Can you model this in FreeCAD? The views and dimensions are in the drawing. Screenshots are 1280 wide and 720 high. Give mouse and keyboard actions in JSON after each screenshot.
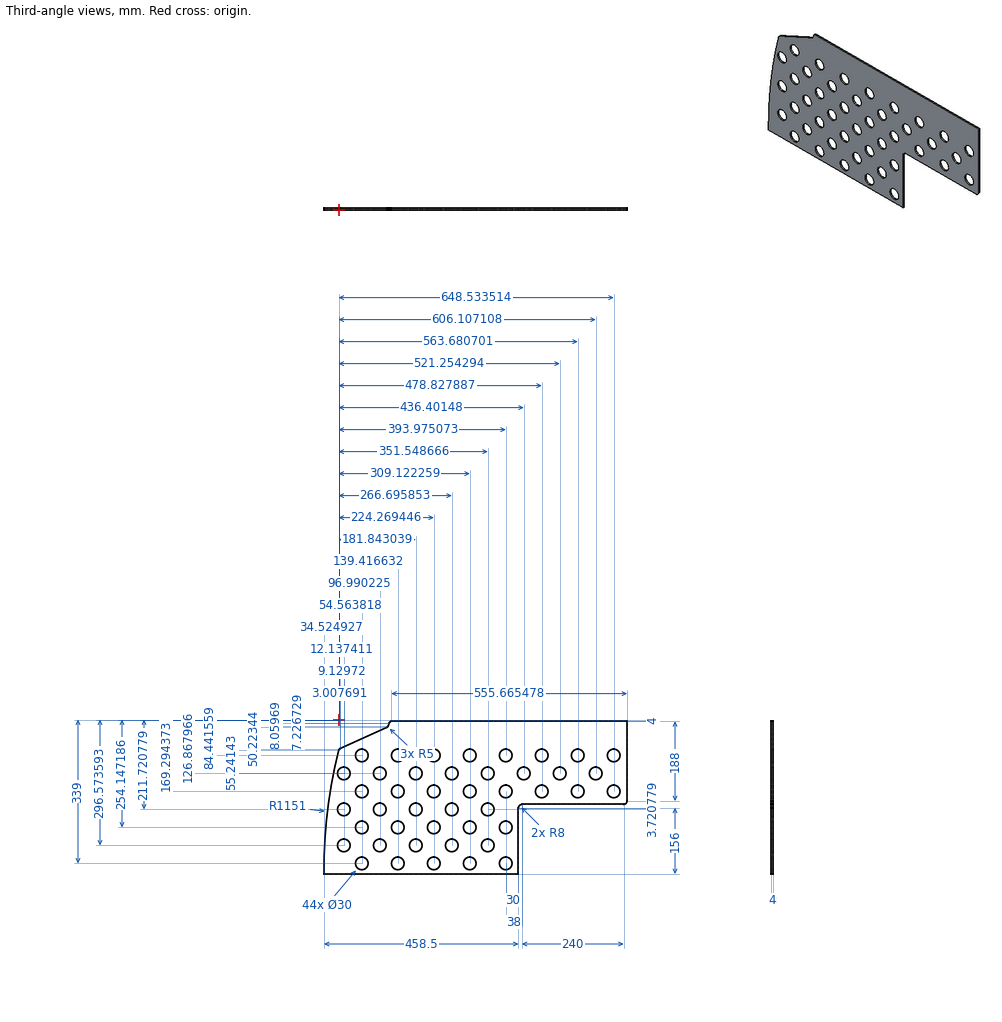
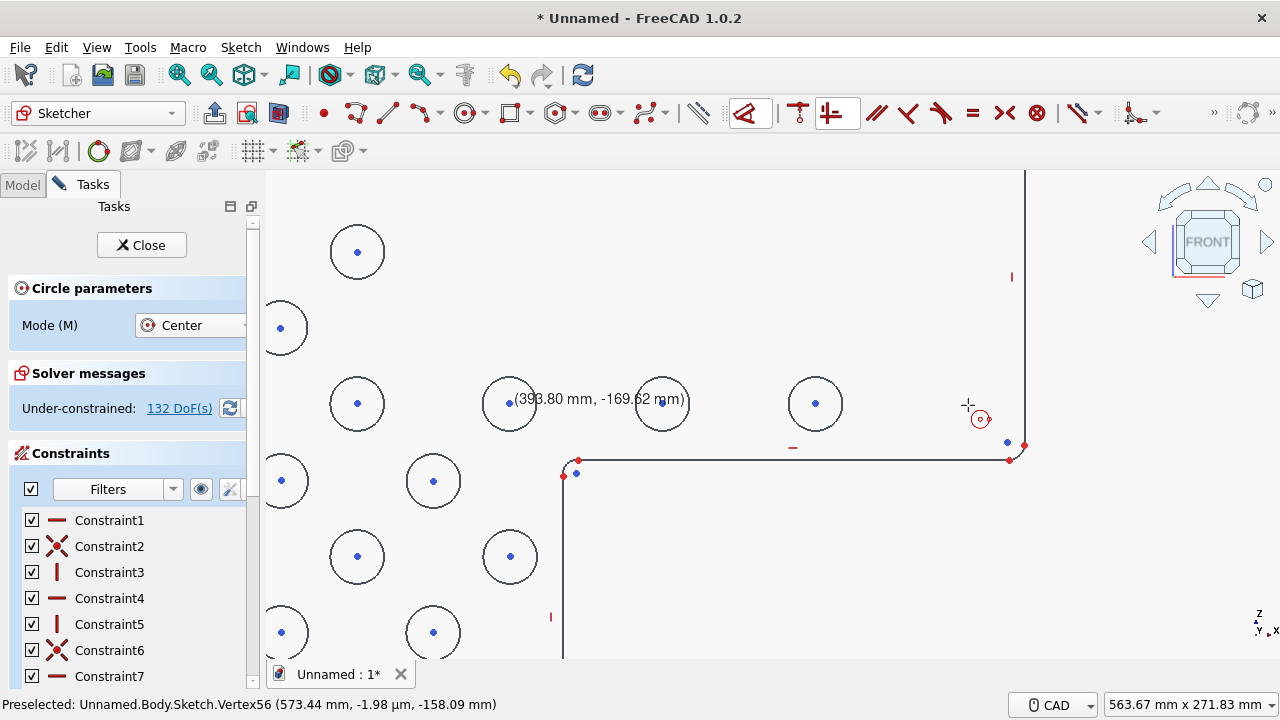
{"action": "left_click", "coordinate": [968, 403]}
{"action": "left_click", "coordinate": [987, 384]}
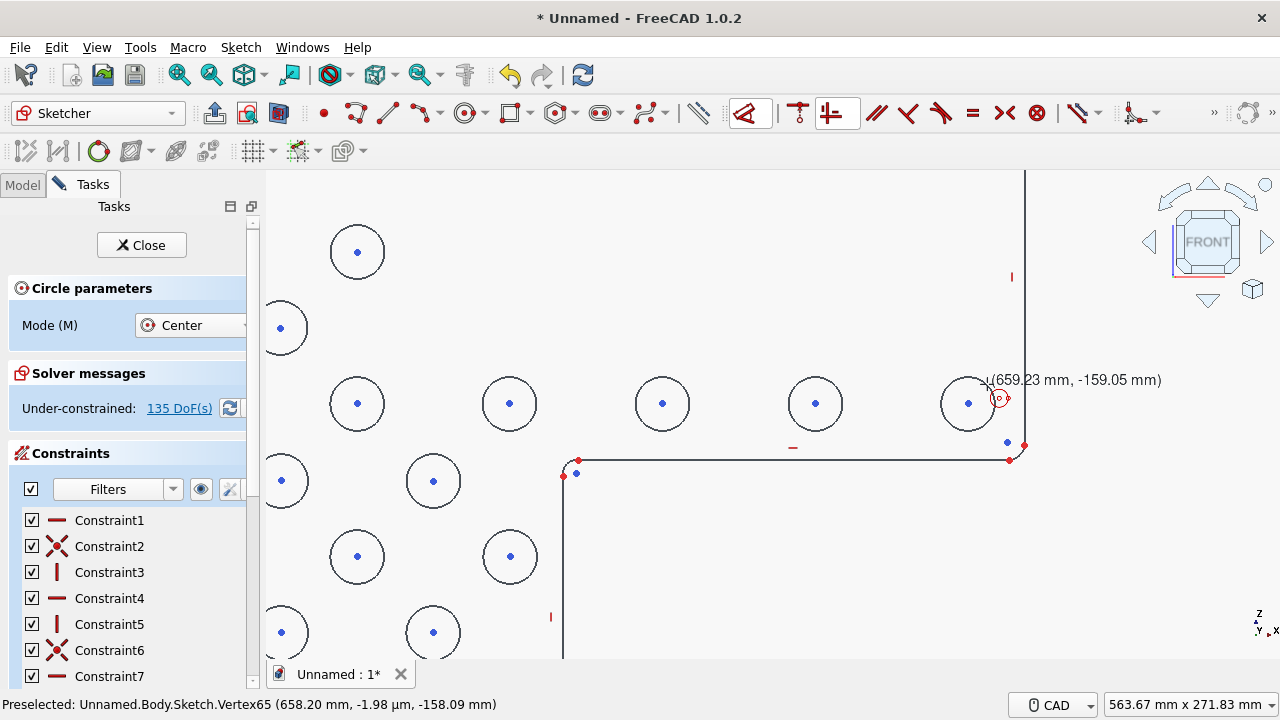
{"action": "left_click", "coordinate": [434, 327]}
{"action": "left_click", "coordinate": [453, 308]}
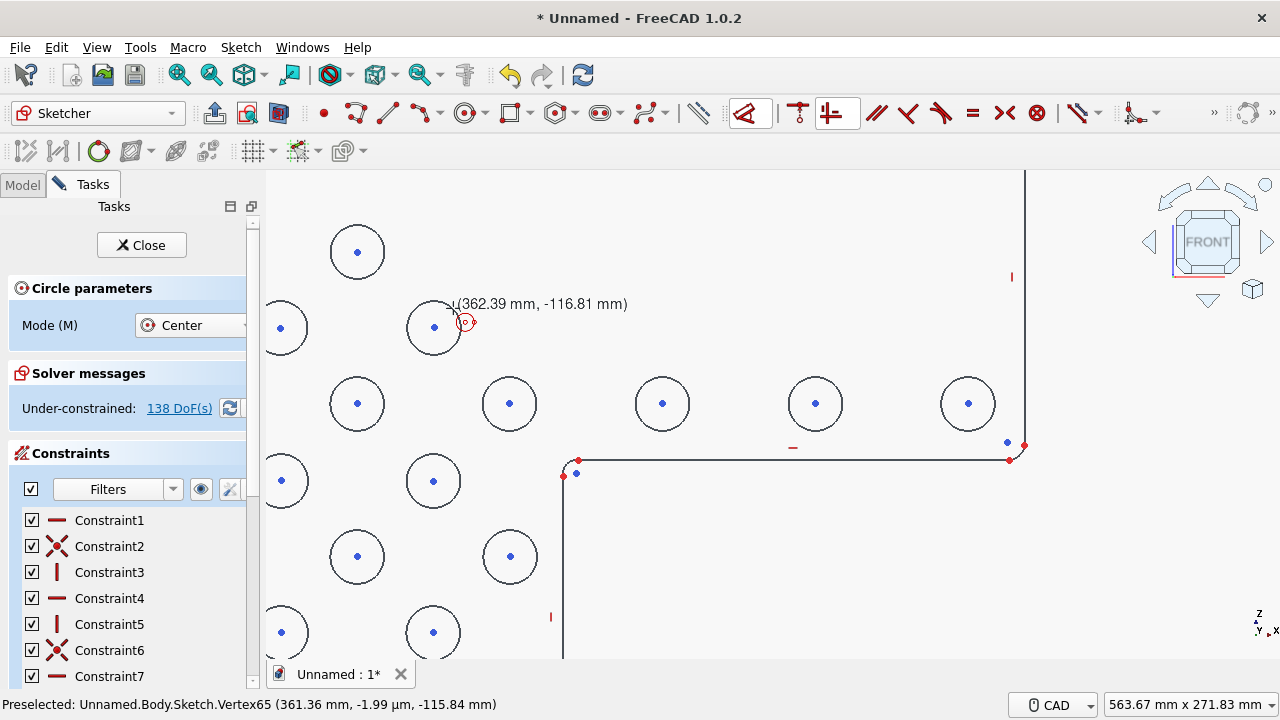
{"action": "left_click", "coordinate": [586, 327]}
{"action": "left_click", "coordinate": [605, 308]}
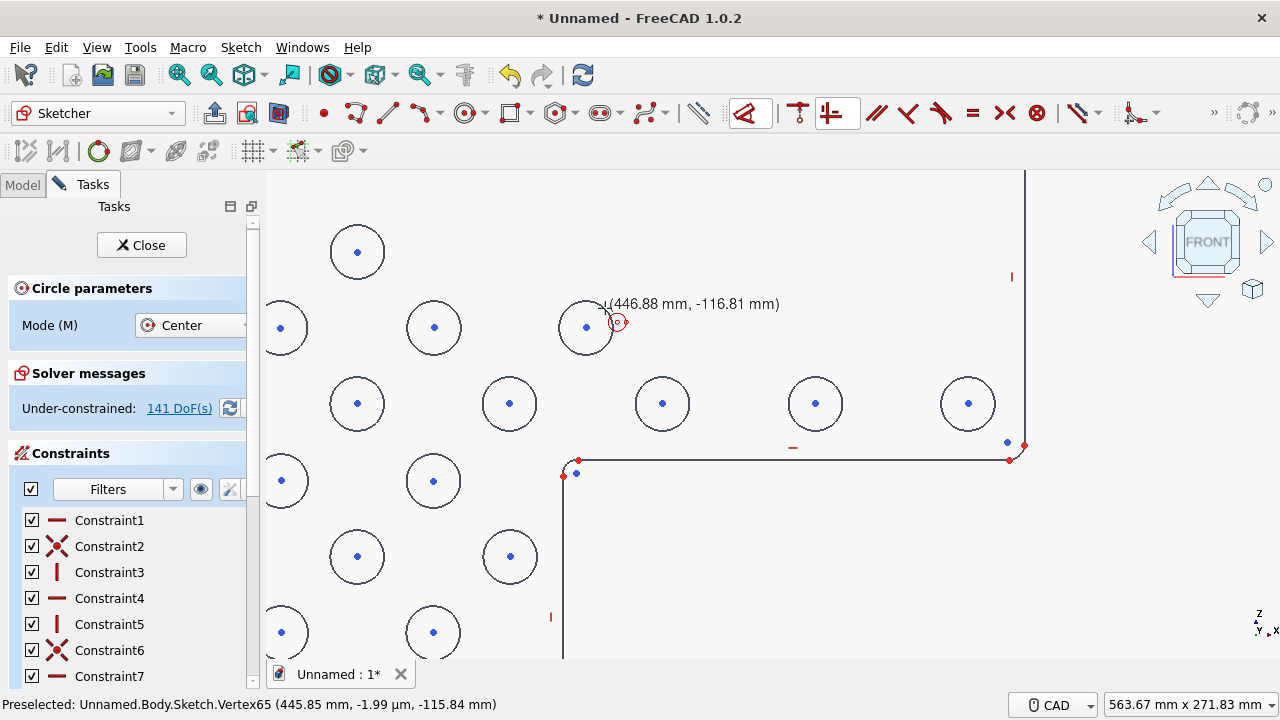
{"action": "left_click", "coordinate": [510, 251]}
{"action": "left_click", "coordinate": [529, 232]}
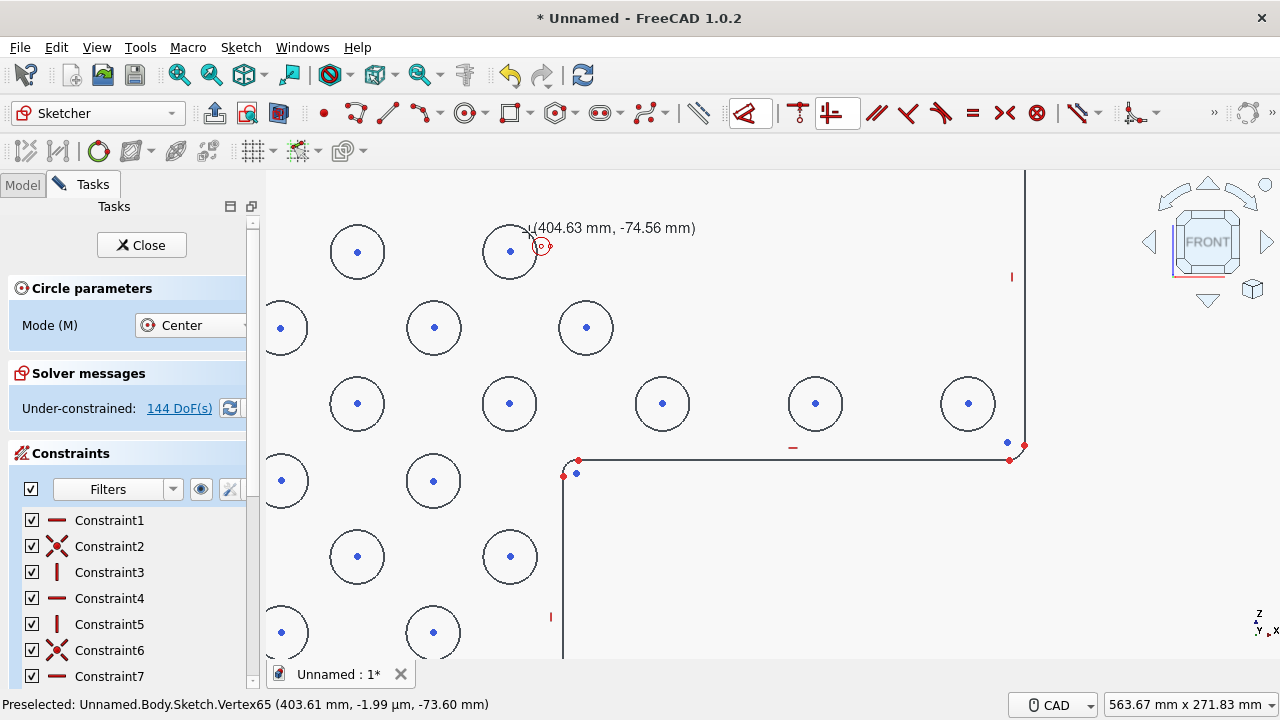
{"action": "left_click", "coordinate": [662, 251]}
{"action": "left_click", "coordinate": [682, 232]}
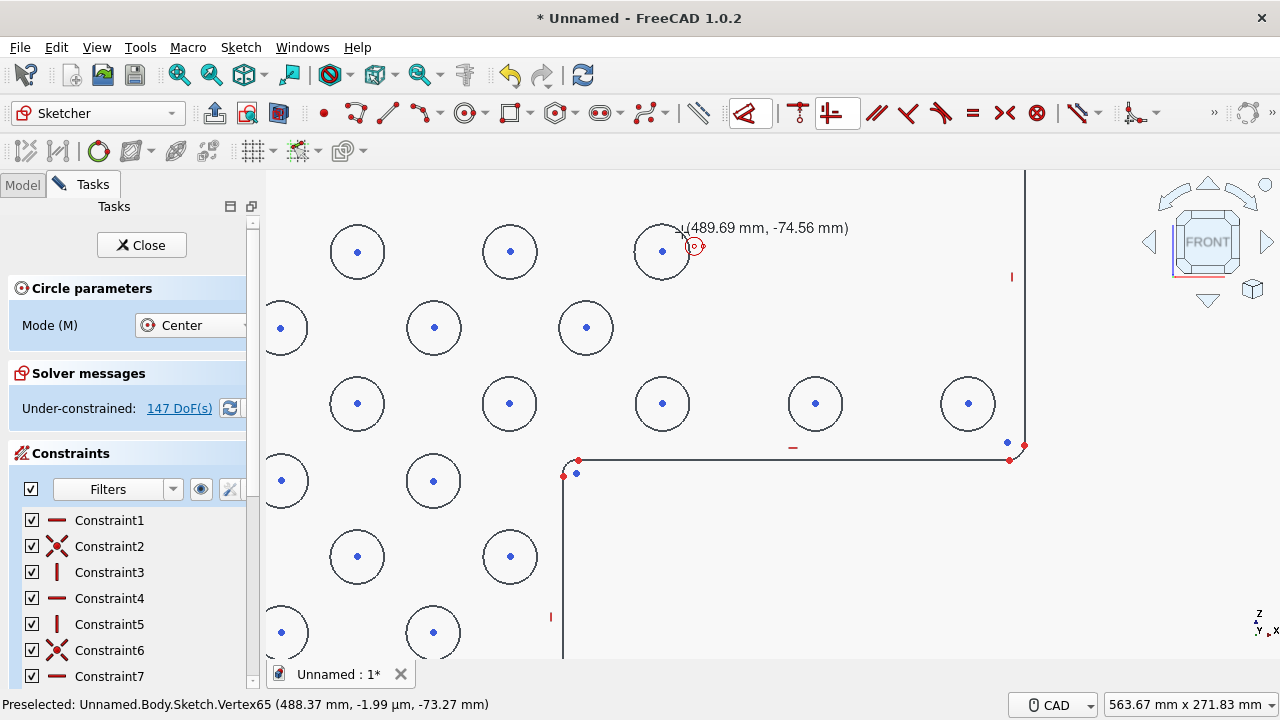
{"action": "left_click", "coordinate": [739, 327]}
{"action": "left_click", "coordinate": [758, 308]}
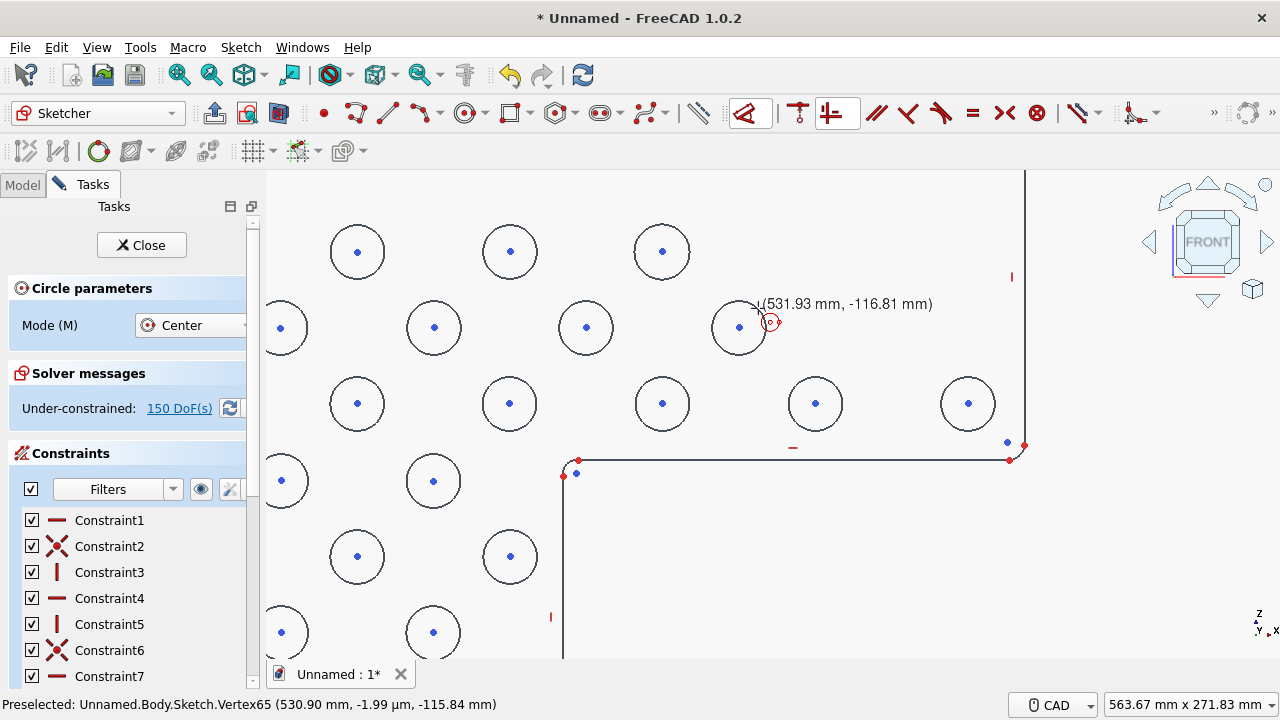
{"action": "left_click", "coordinate": [891, 327]}
{"action": "left_click", "coordinate": [911, 308]}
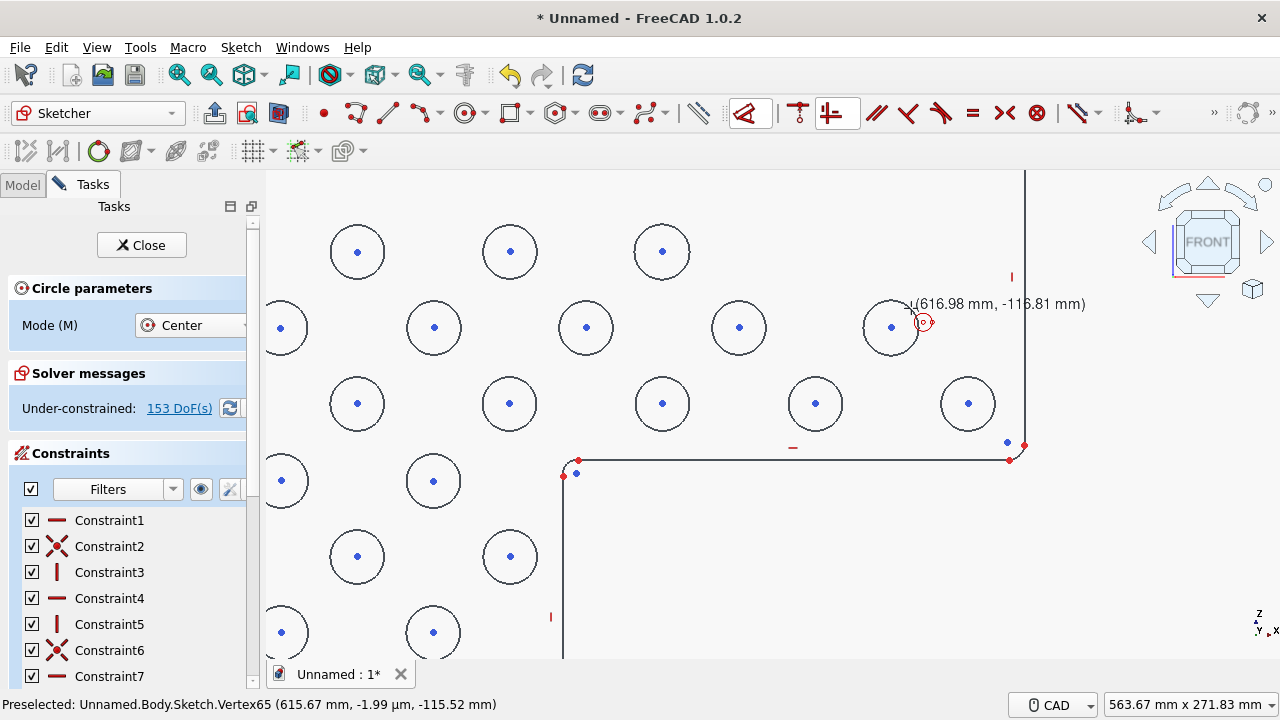
{"action": "left_click", "coordinate": [815, 251]}
{"action": "left_click", "coordinate": [834, 232]}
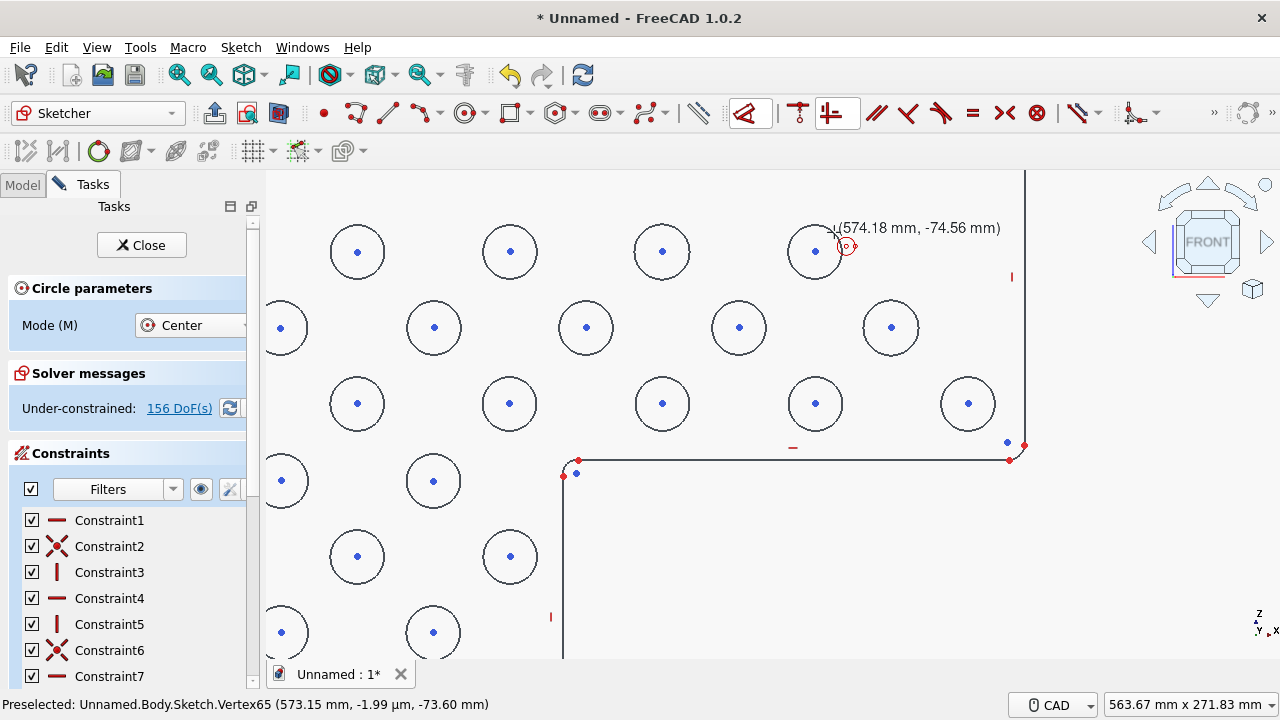
{"action": "left_click", "coordinate": [968, 251]}
{"action": "left_click", "coordinate": [987, 232]}
{"action": "key", "text": "Escape"}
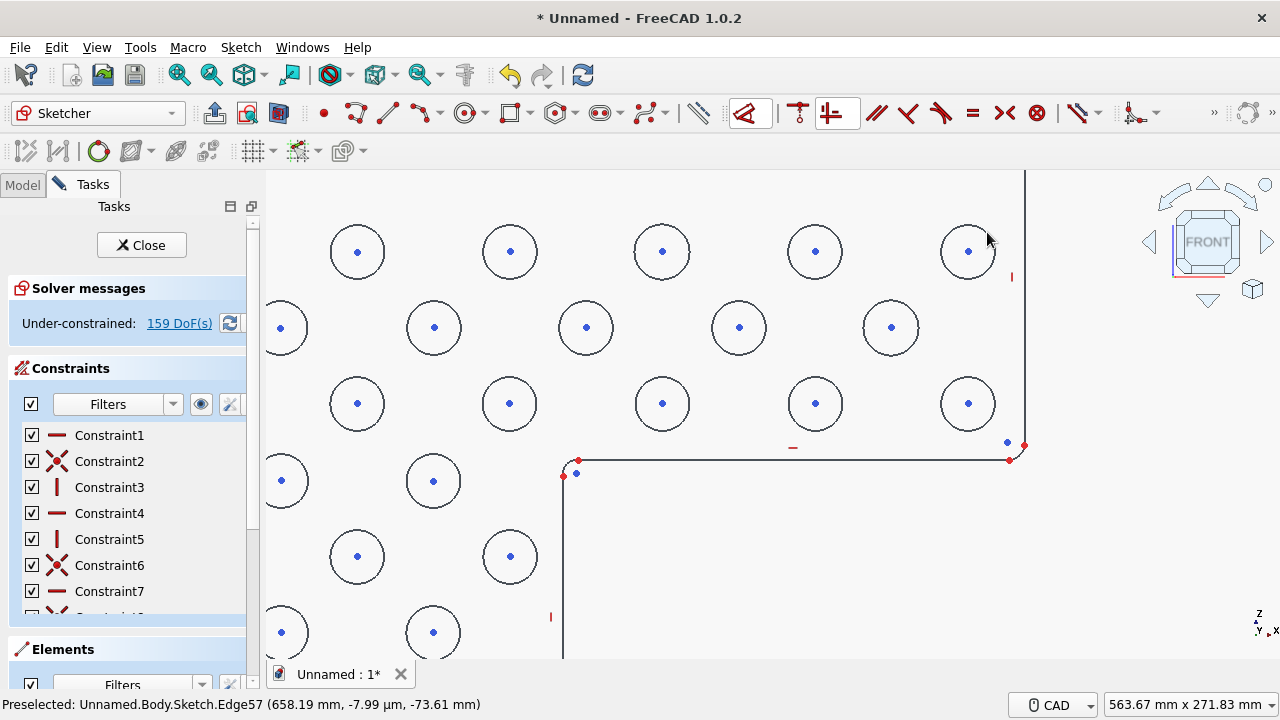
{"action": "scroll", "coordinate": [968, 405], "scroll_direction": "down", "scroll_amount": 4}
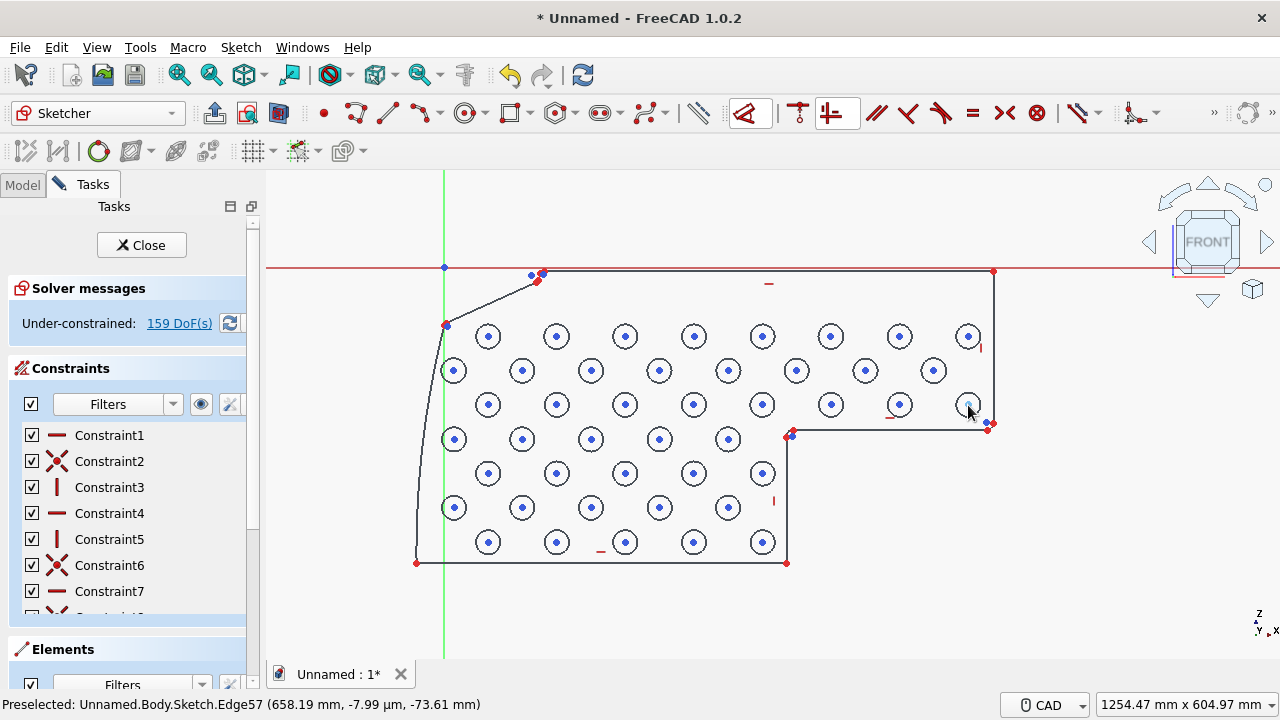
{"action": "scroll", "coordinate": [540, 277], "scroll_direction": "up", "scroll_amount": 7}